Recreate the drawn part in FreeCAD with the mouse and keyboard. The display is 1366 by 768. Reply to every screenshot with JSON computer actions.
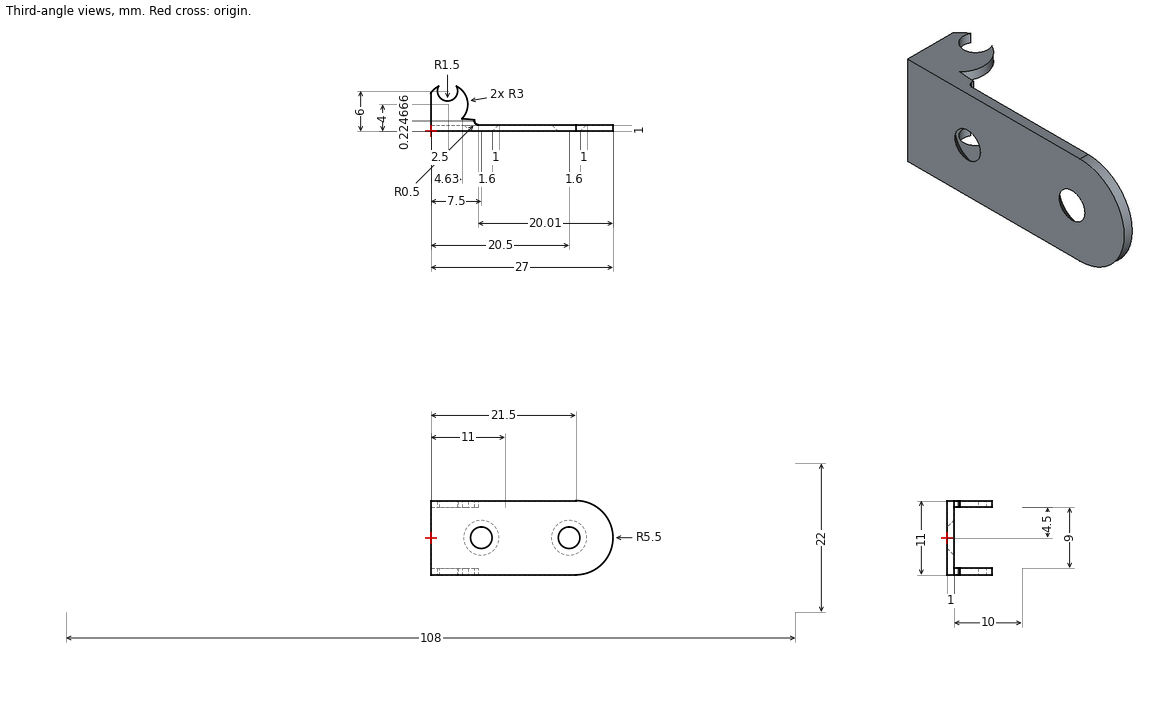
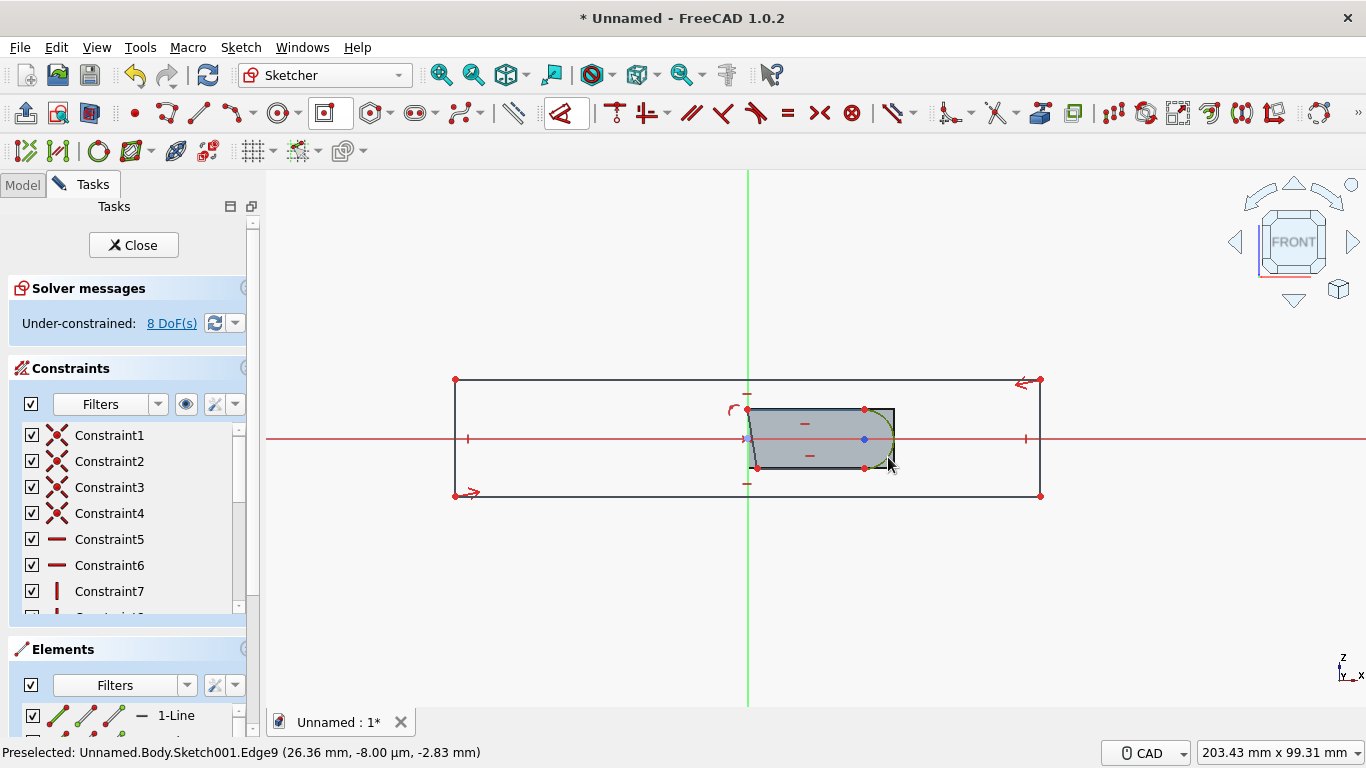
{"action": "key", "text": "t"}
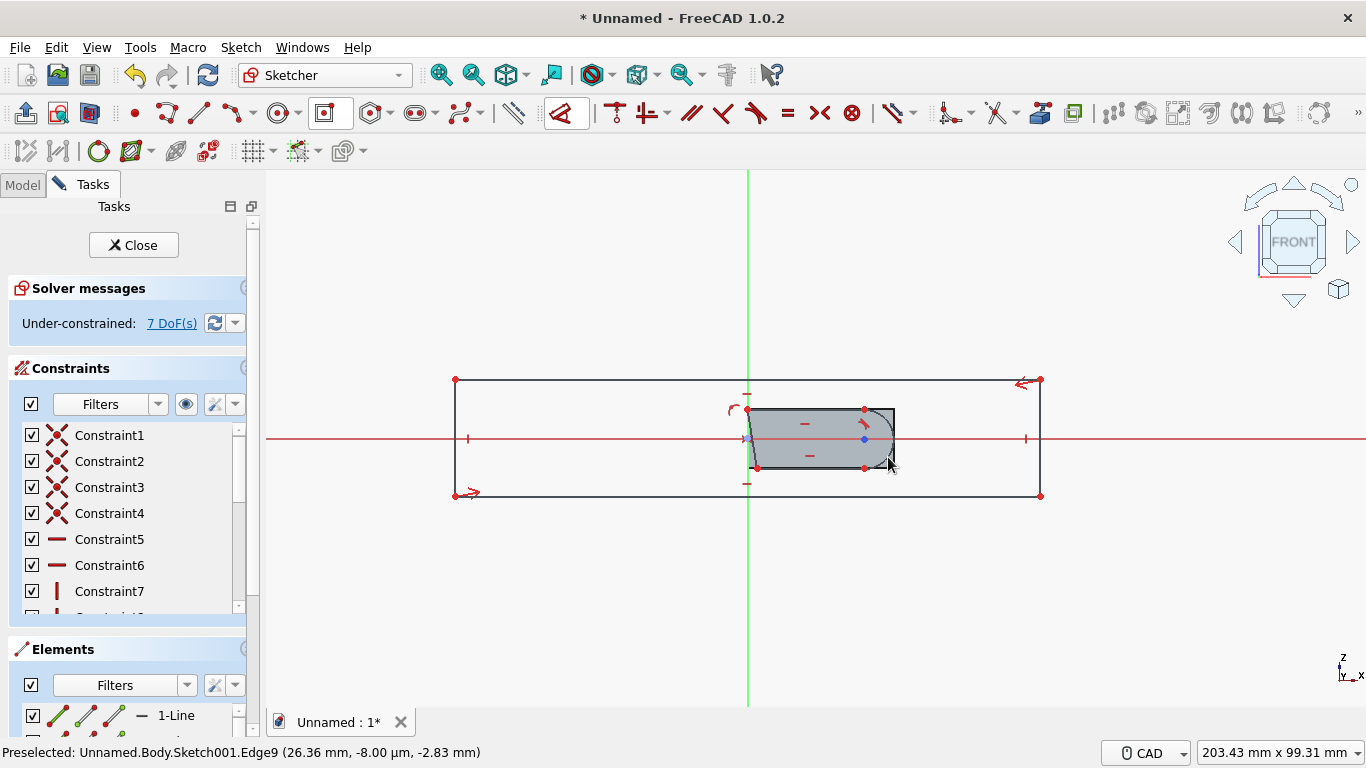
{"action": "left_click", "coordinate": [789, 469]}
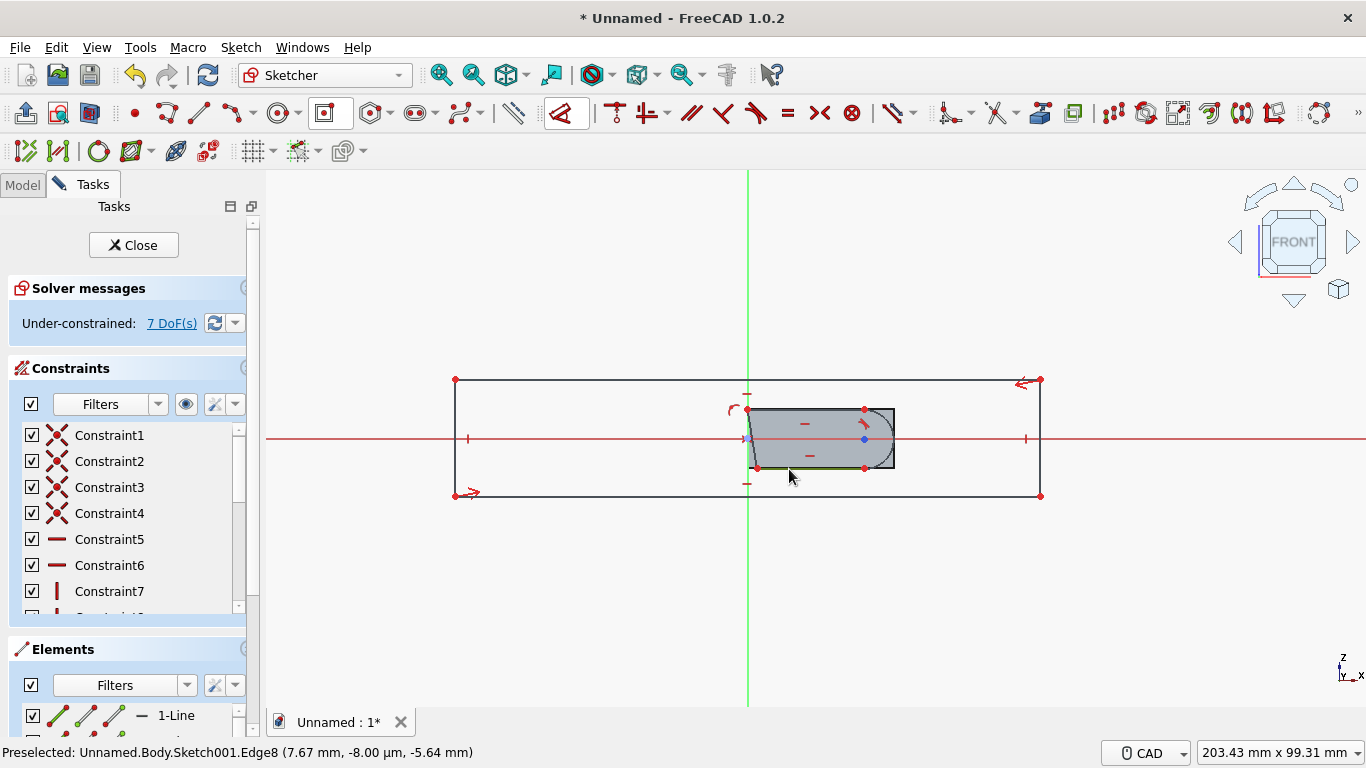
{"action": "left_click", "coordinate": [888, 457]}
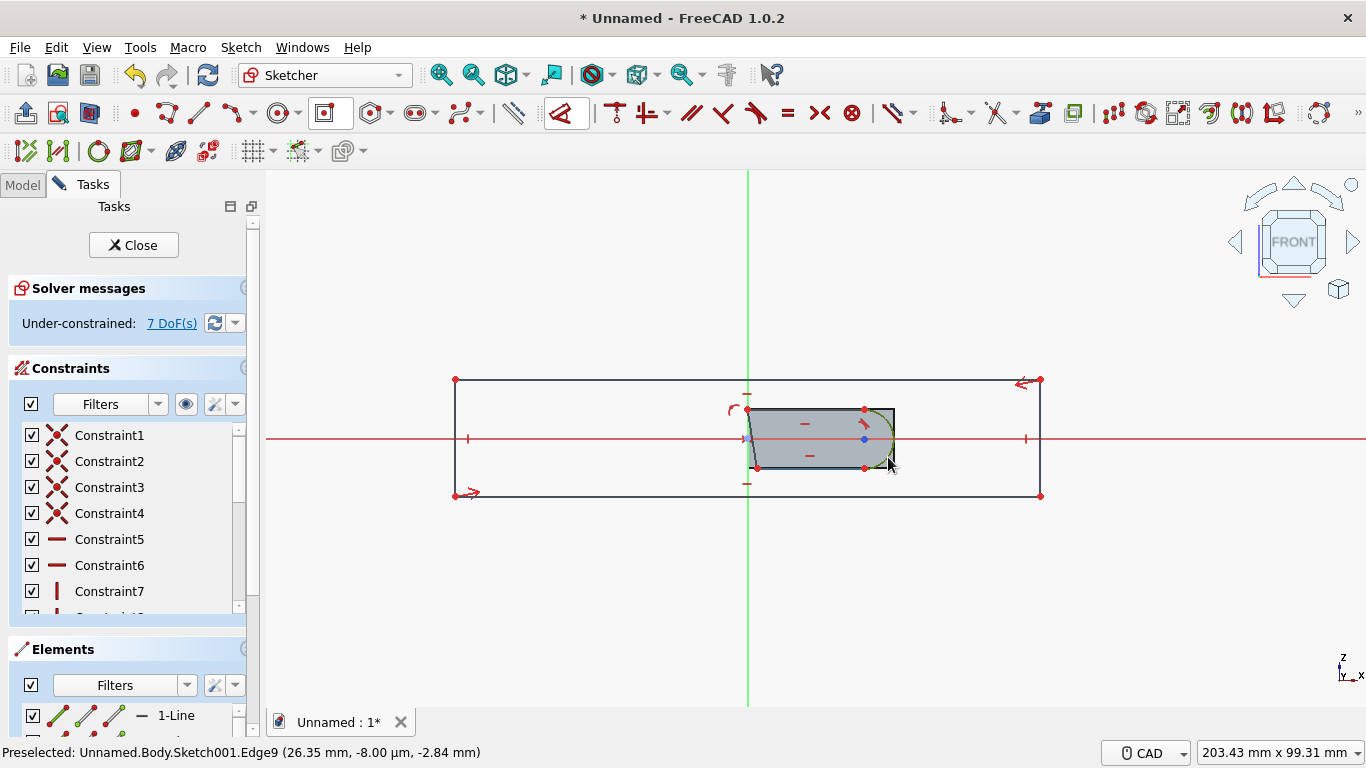
{"action": "key", "text": "t"}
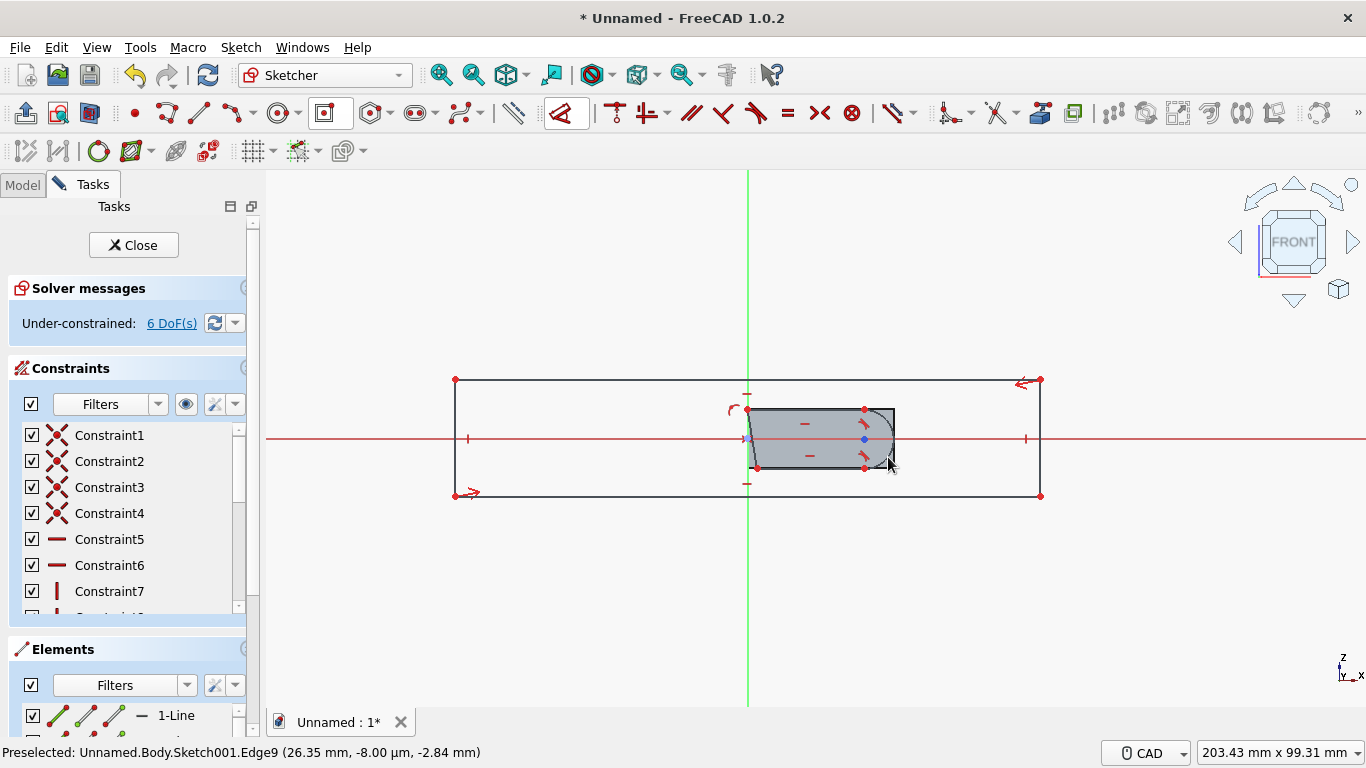
{"action": "scroll", "coordinate": [750, 428], "scroll_direction": "up", "scroll_amount": 2}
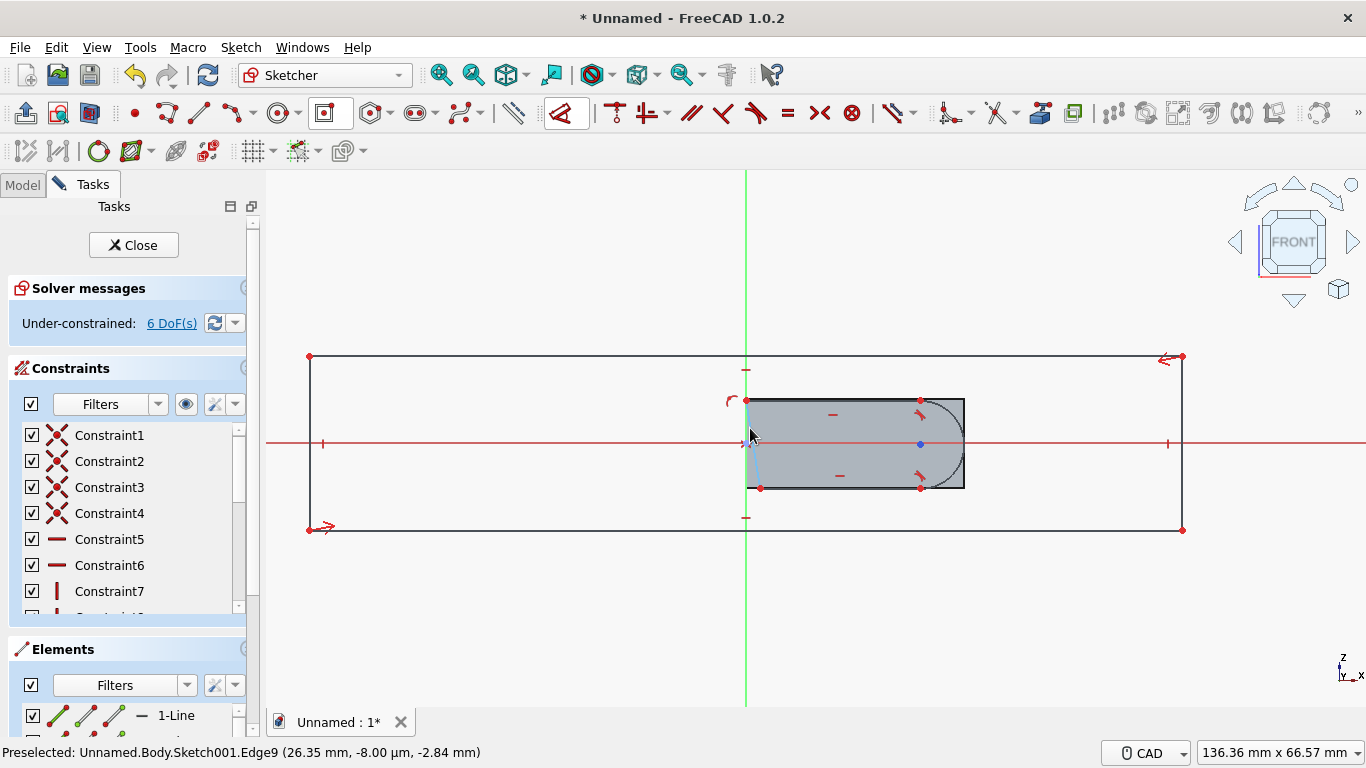
{"action": "left_click", "coordinate": [750, 427]}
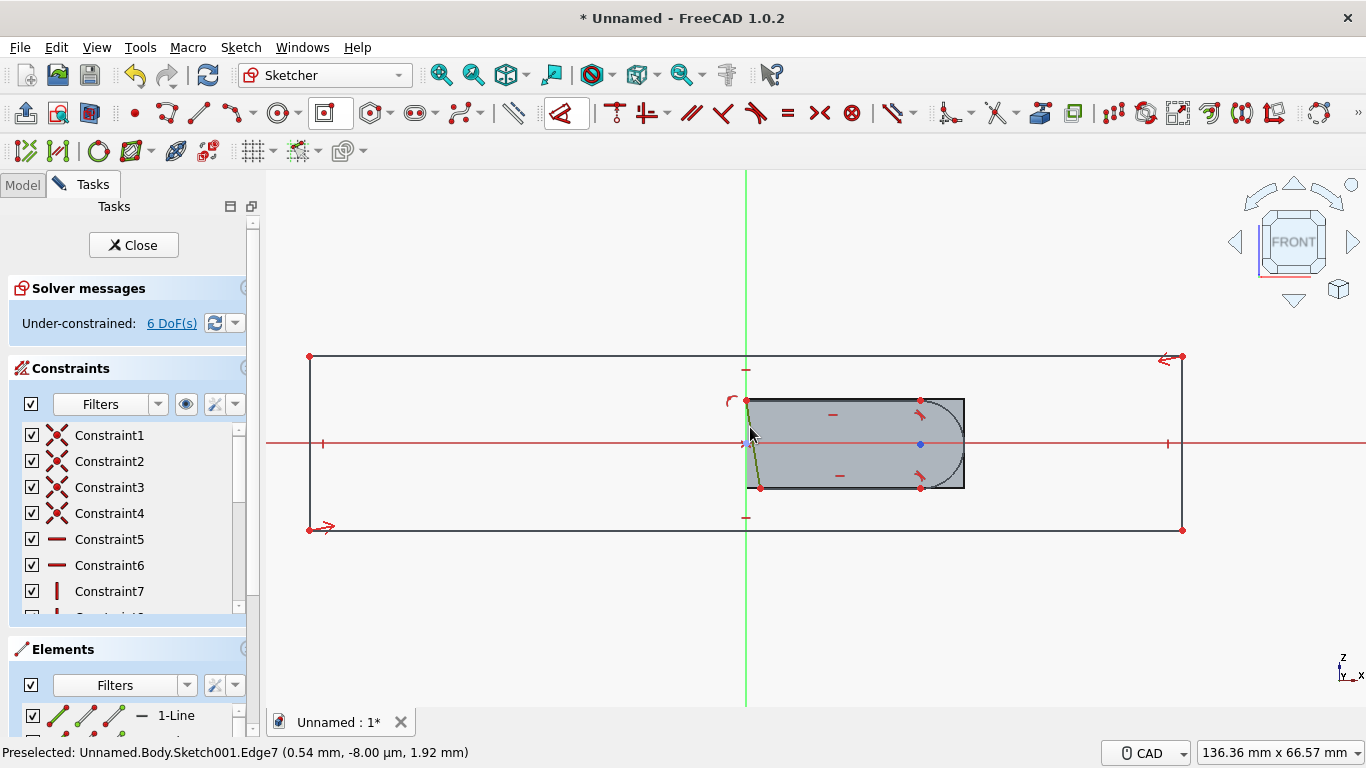
{"action": "key", "text": "v"}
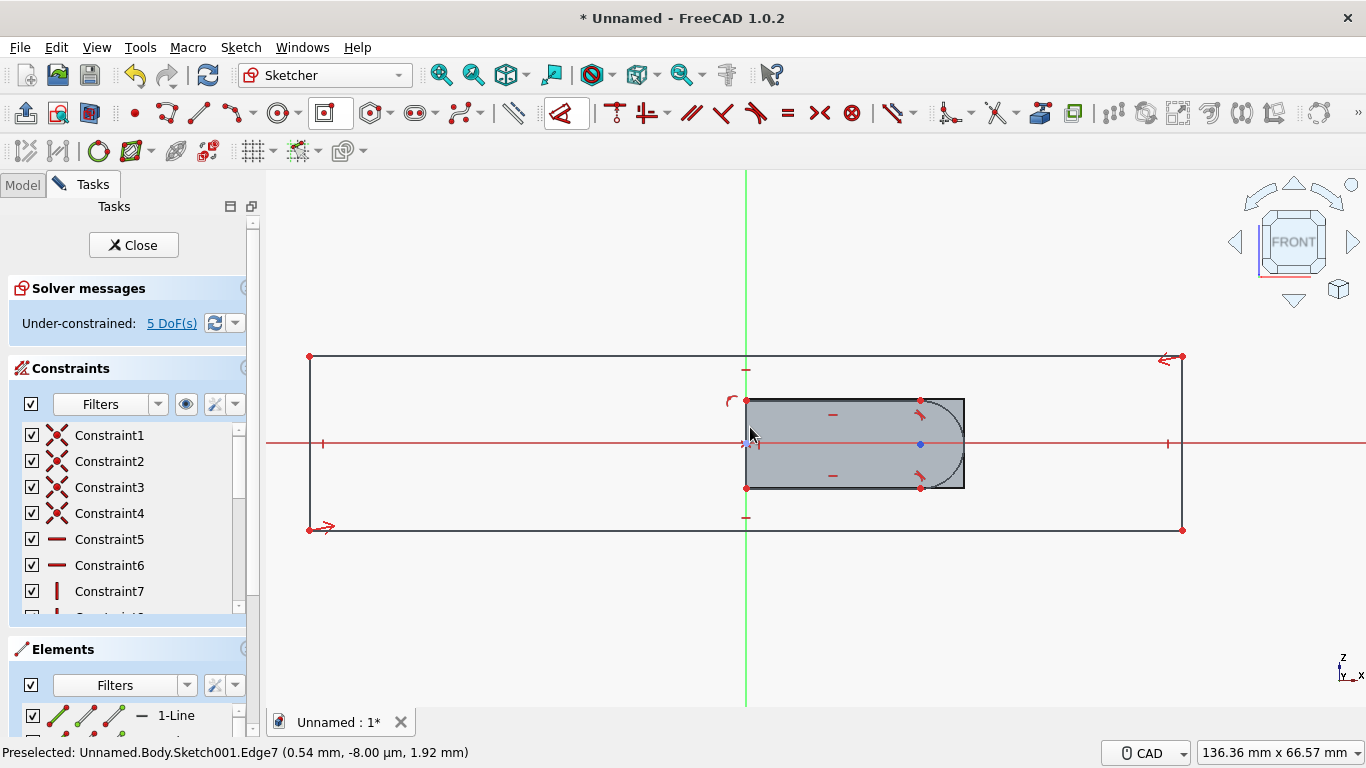
{"action": "left_click", "coordinate": [920, 445]}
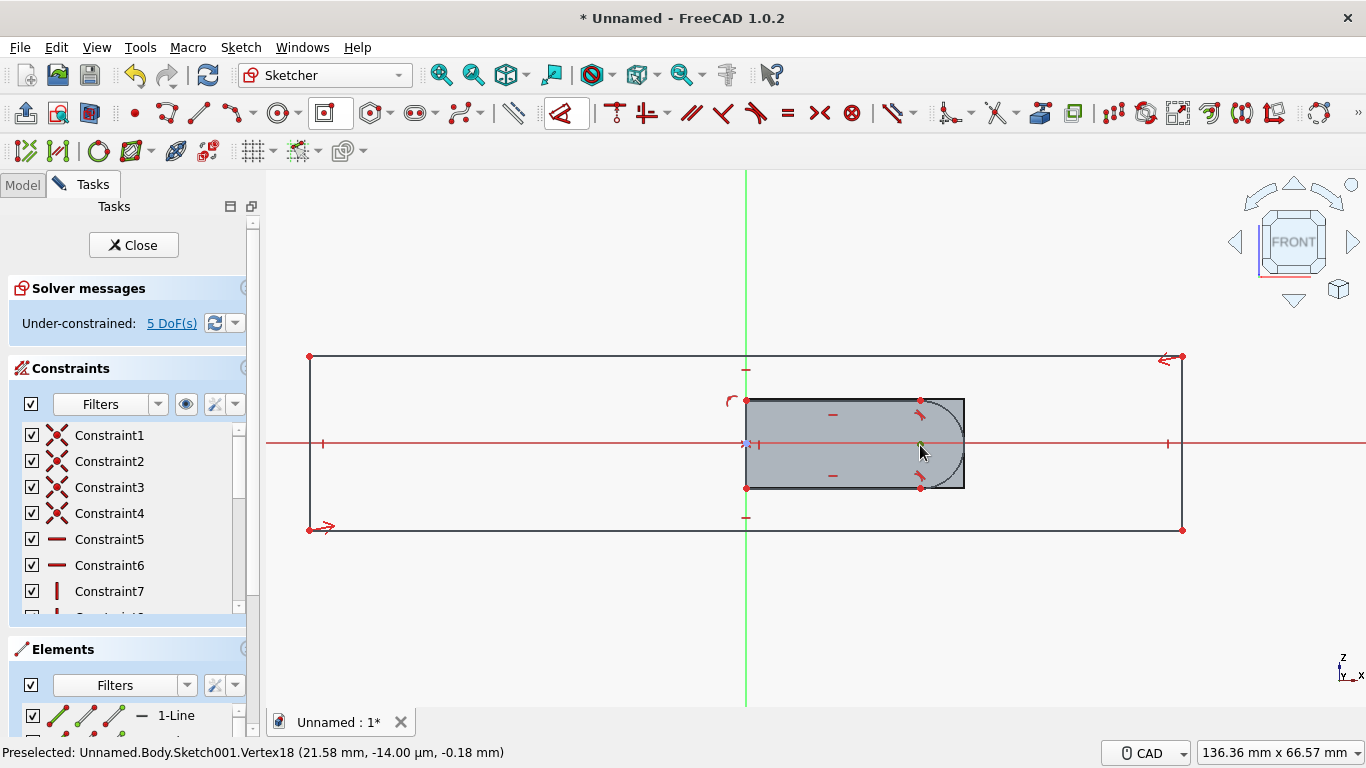
{"action": "left_click", "coordinate": [359, 443]}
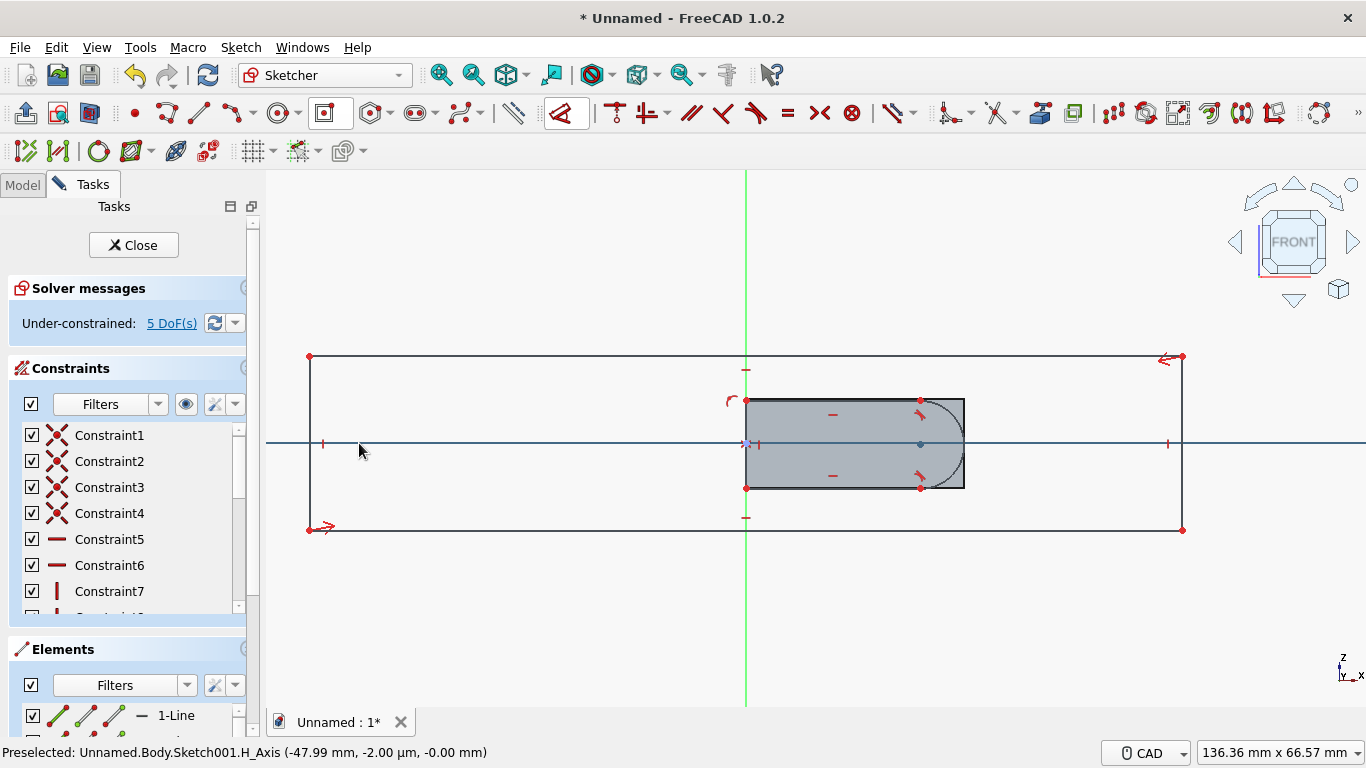
{"action": "key", "text": "c"}